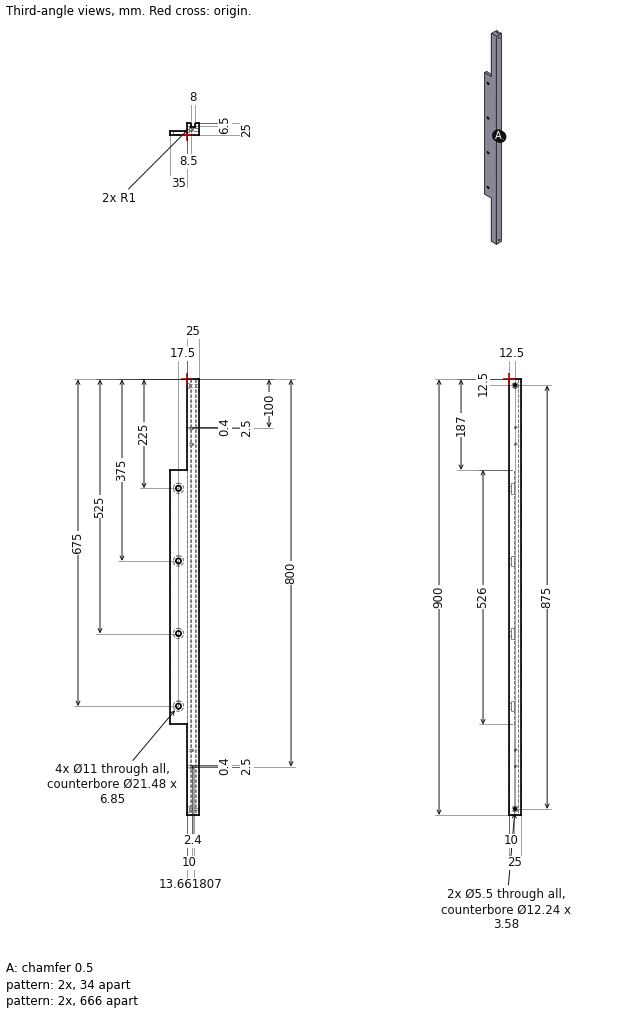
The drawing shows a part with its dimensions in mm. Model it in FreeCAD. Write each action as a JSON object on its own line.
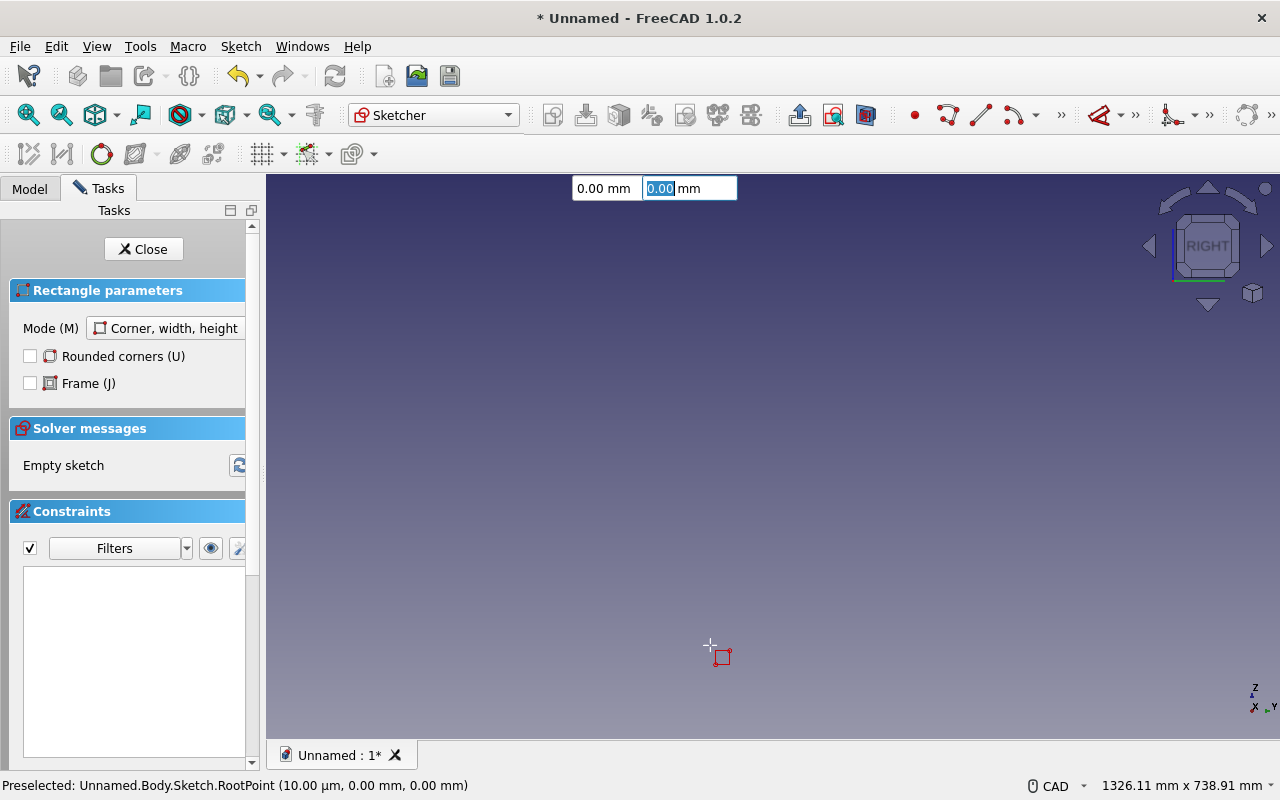
{"action": "left_click", "coordinate": [709, 645]}
{"action": "key", "text": "Escape"}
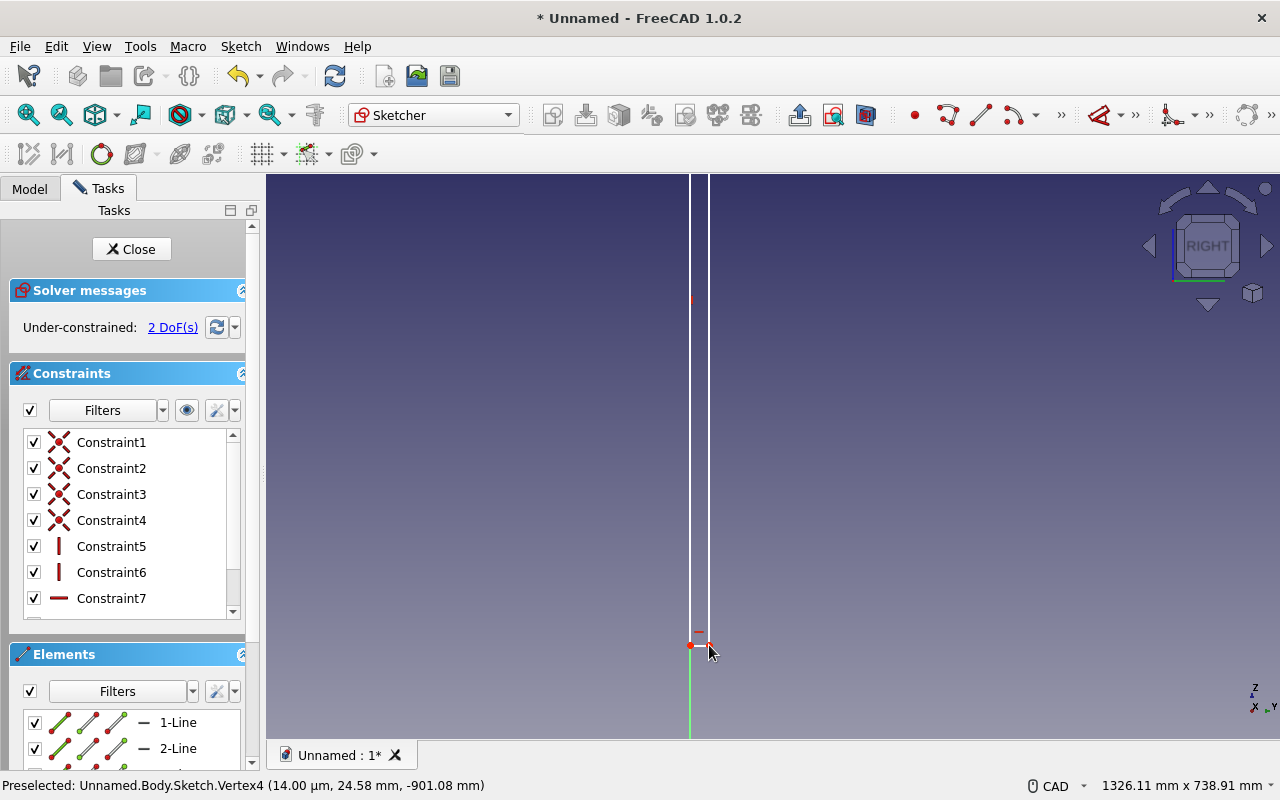
{"action": "scroll", "coordinate": [700, 646], "scroll_direction": "up", "scroll_amount": 4}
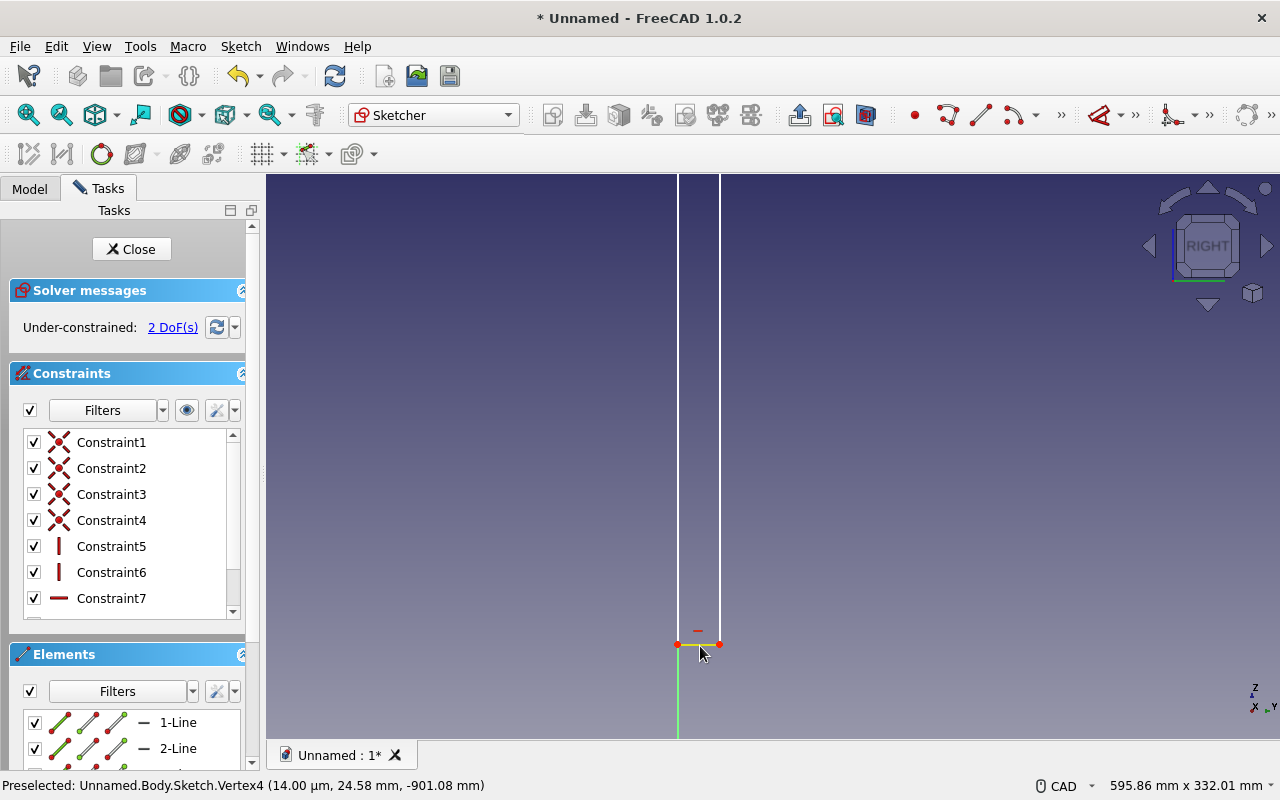
{"action": "left_click", "coordinate": [699, 645]}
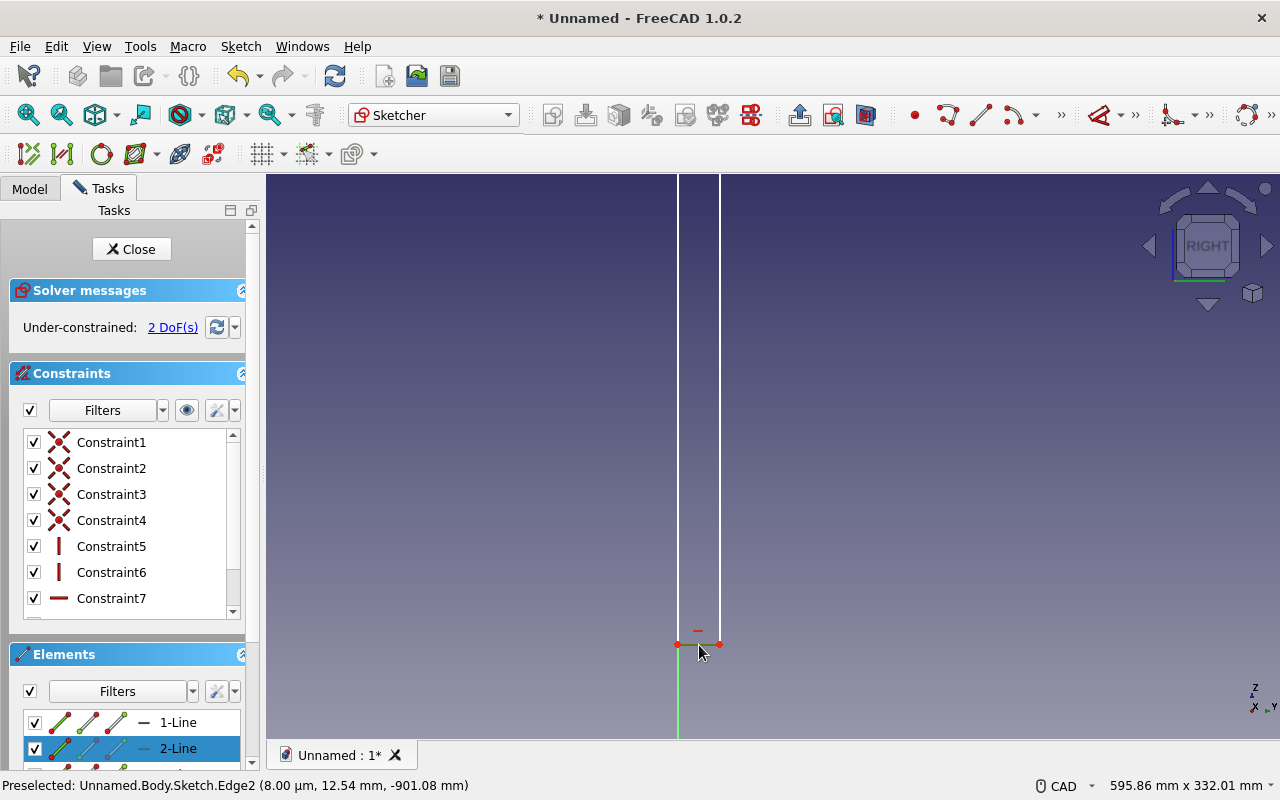
{"action": "key", "text": "l"}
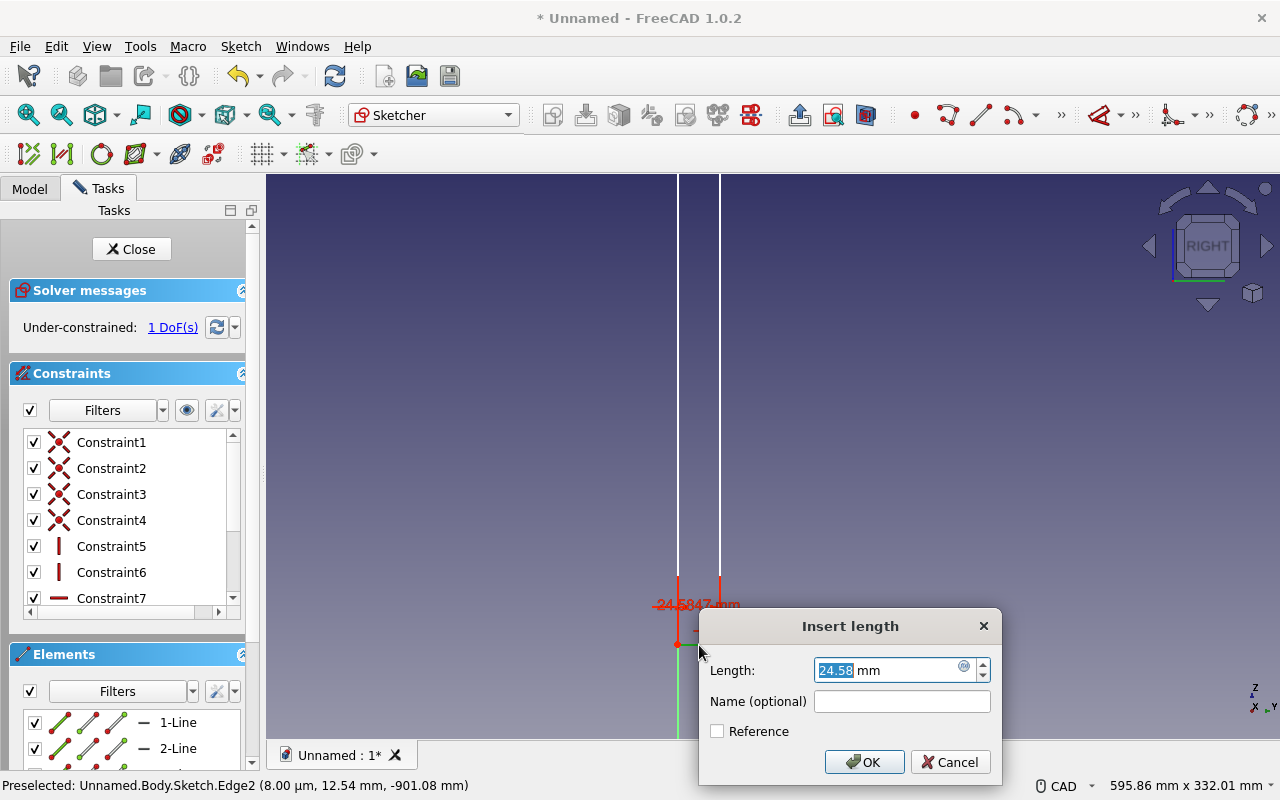
{"action": "type", "text": "25"}
{"action": "key", "text": "Return"}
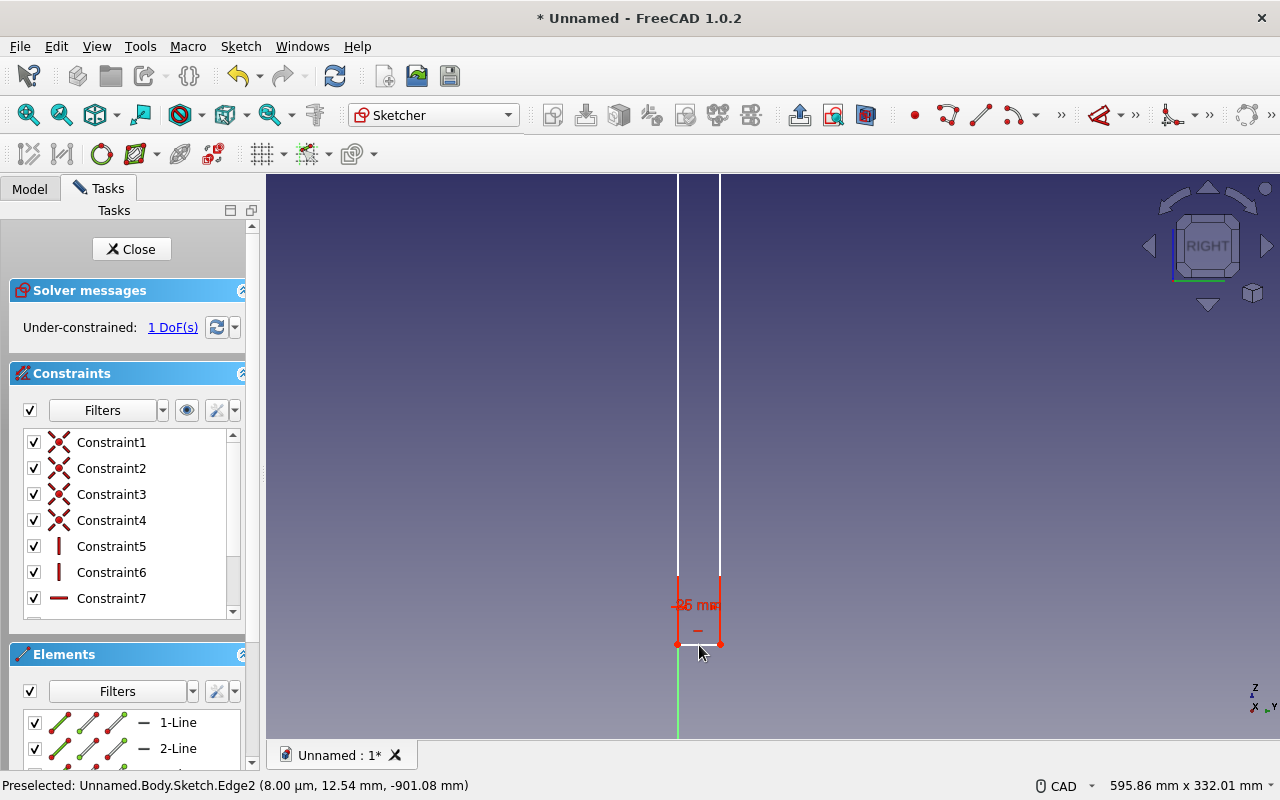
{"action": "scroll", "coordinate": [706, 646], "scroll_direction": "down", "scroll_amount": 7}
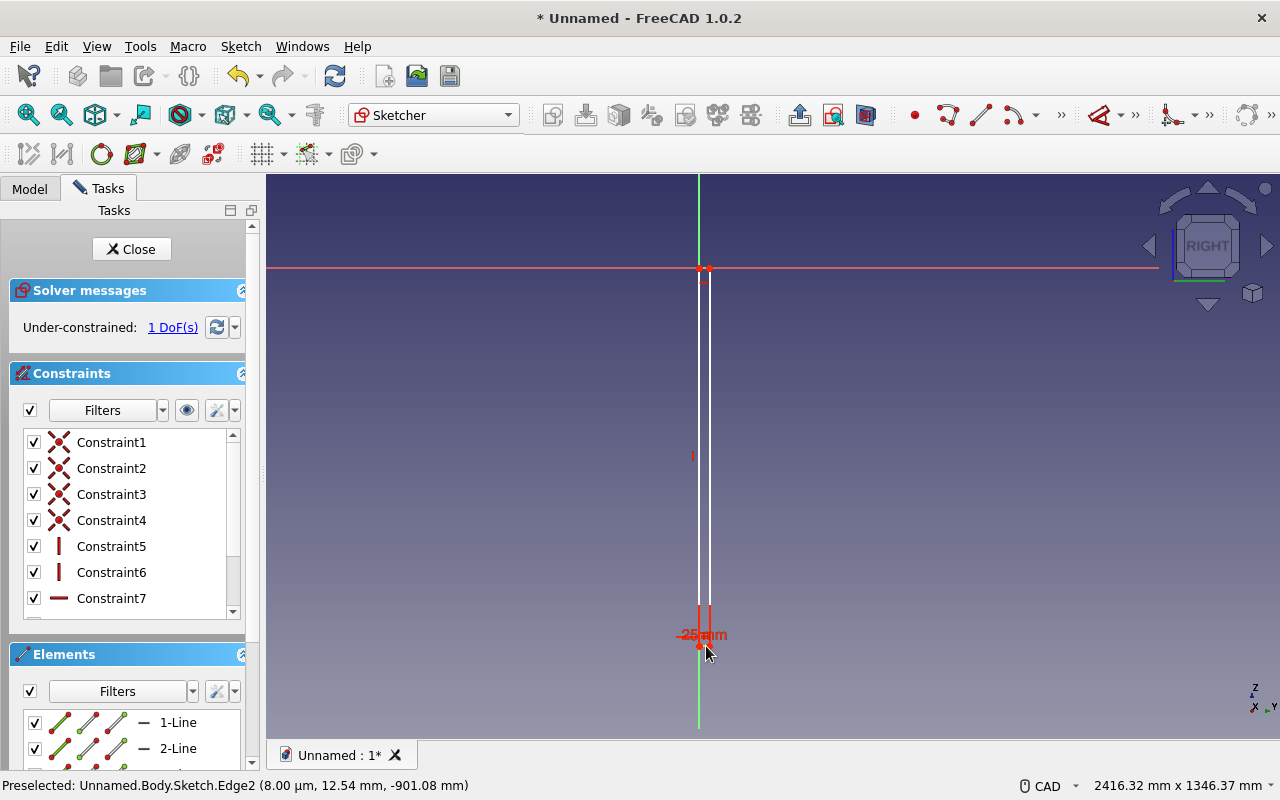
{"action": "scroll", "coordinate": [699, 571], "scroll_direction": "up", "scroll_amount": 2}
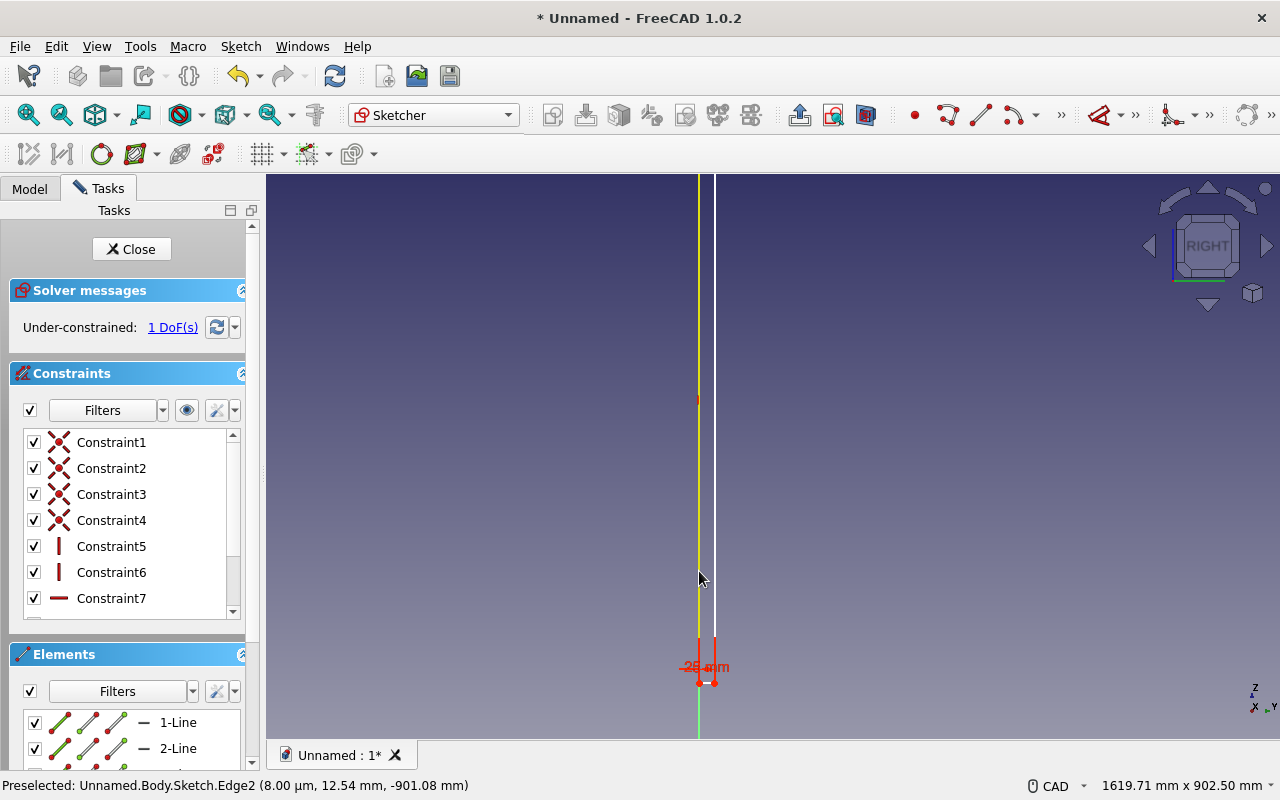
{"action": "left_click", "coordinate": [699, 570]}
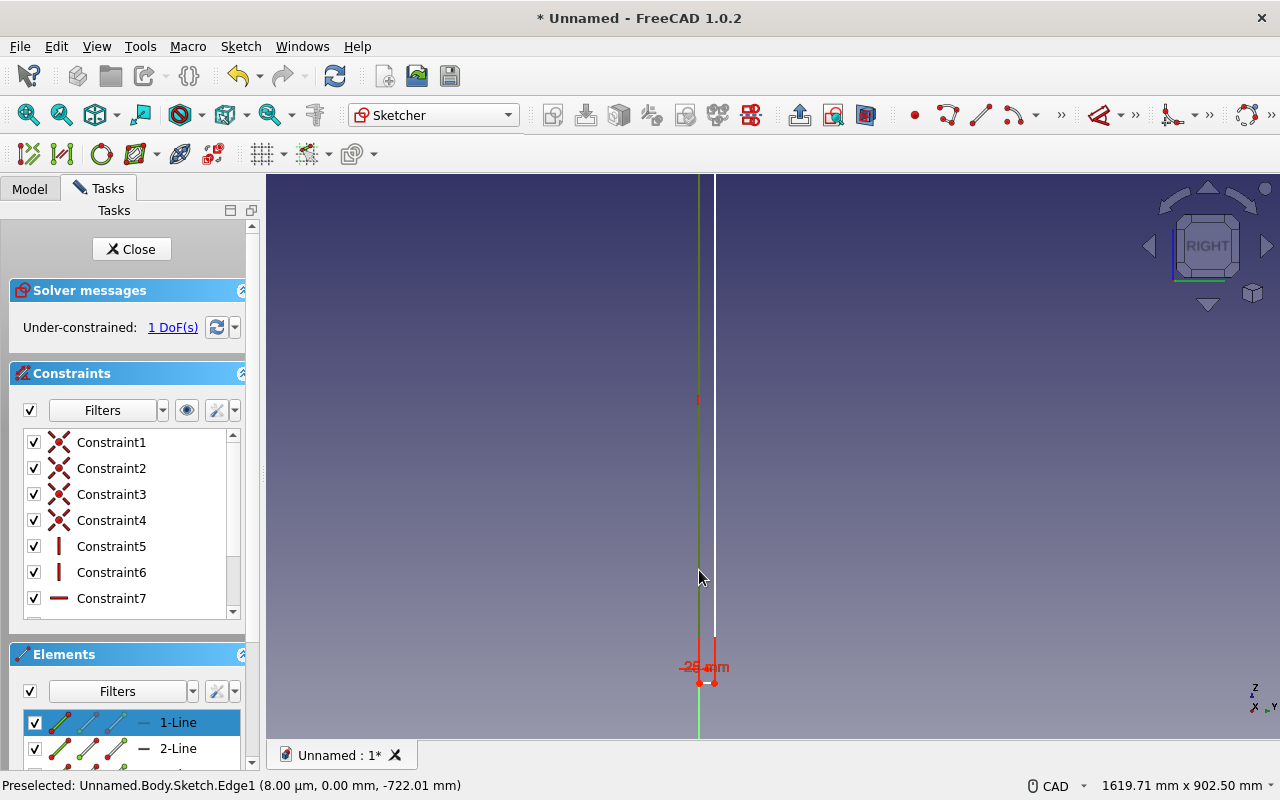
{"action": "key", "text": "i"}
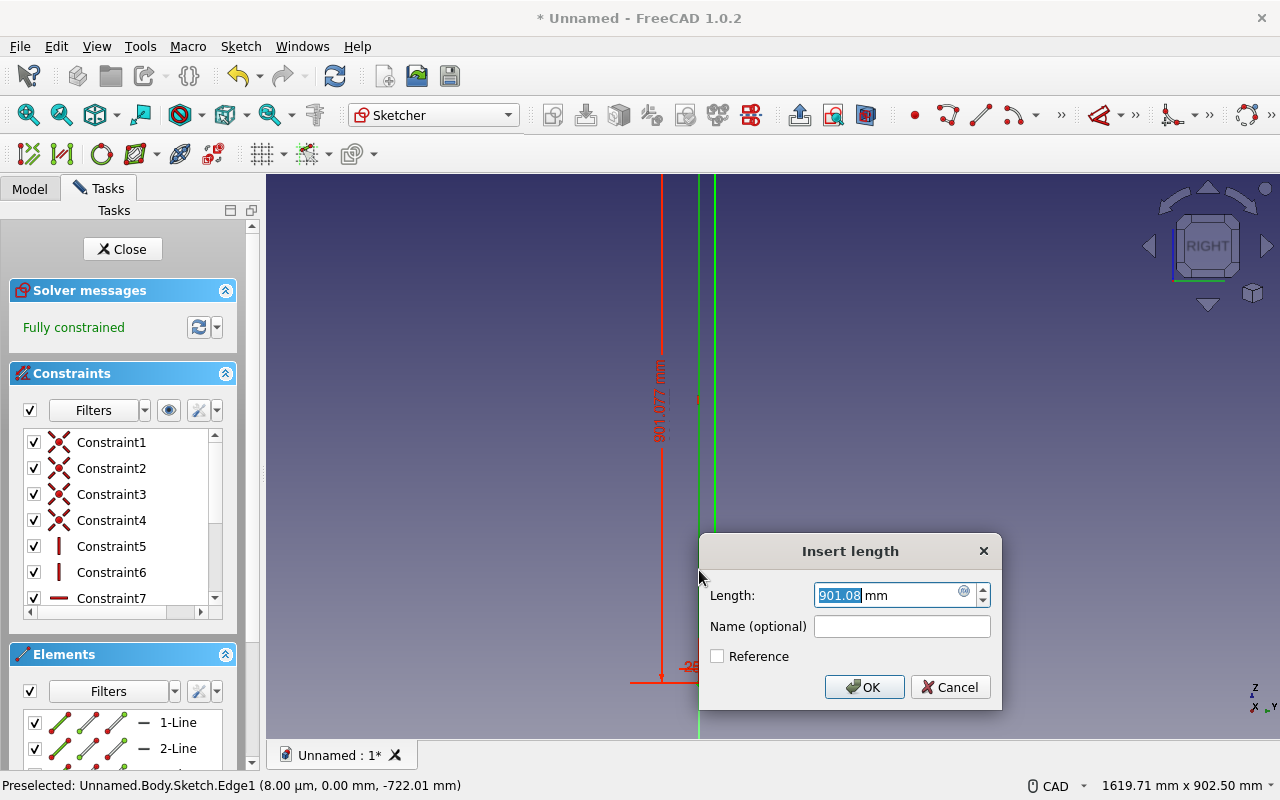
{"action": "type", "text": "900"}
{"action": "key", "text": "Return"}